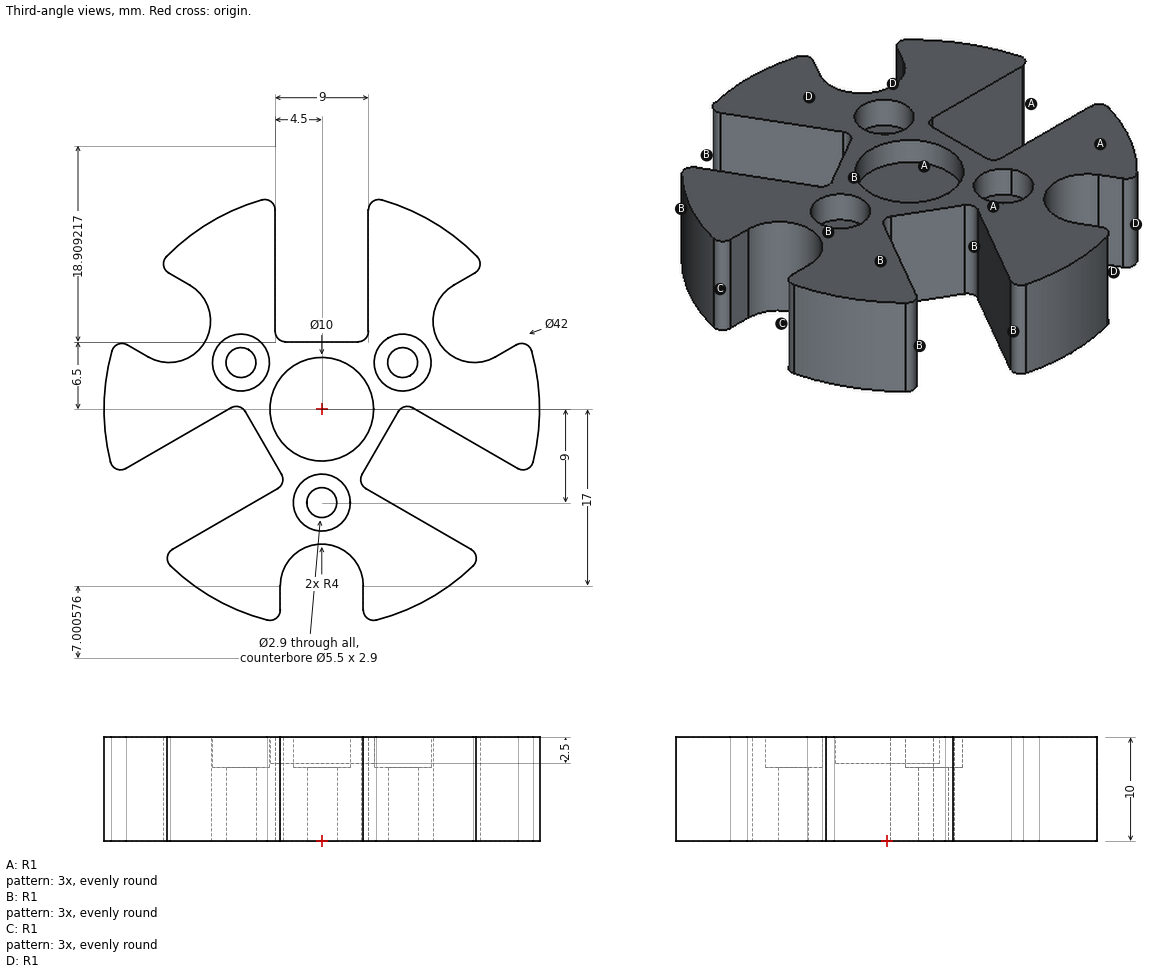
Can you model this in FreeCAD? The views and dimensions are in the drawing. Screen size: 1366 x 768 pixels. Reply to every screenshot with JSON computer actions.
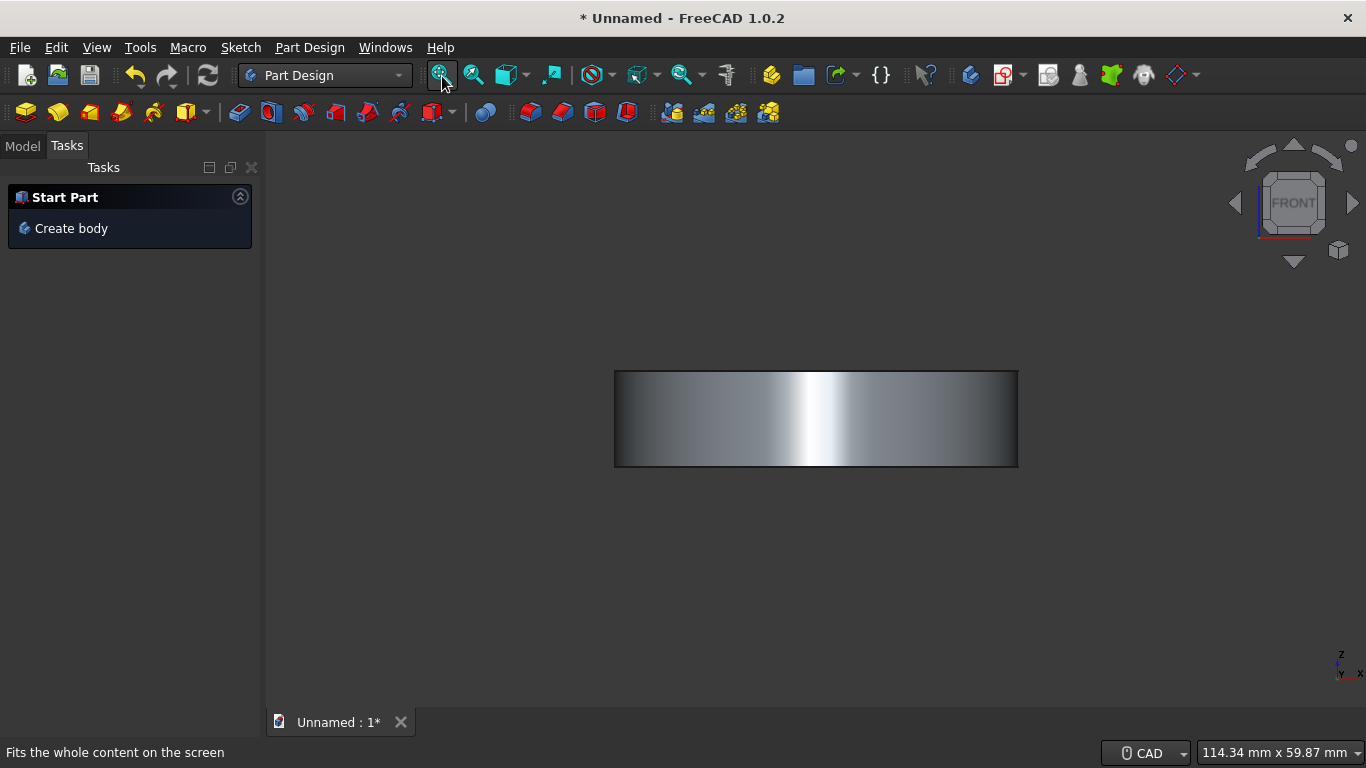
{"action": "key", "text": "3"}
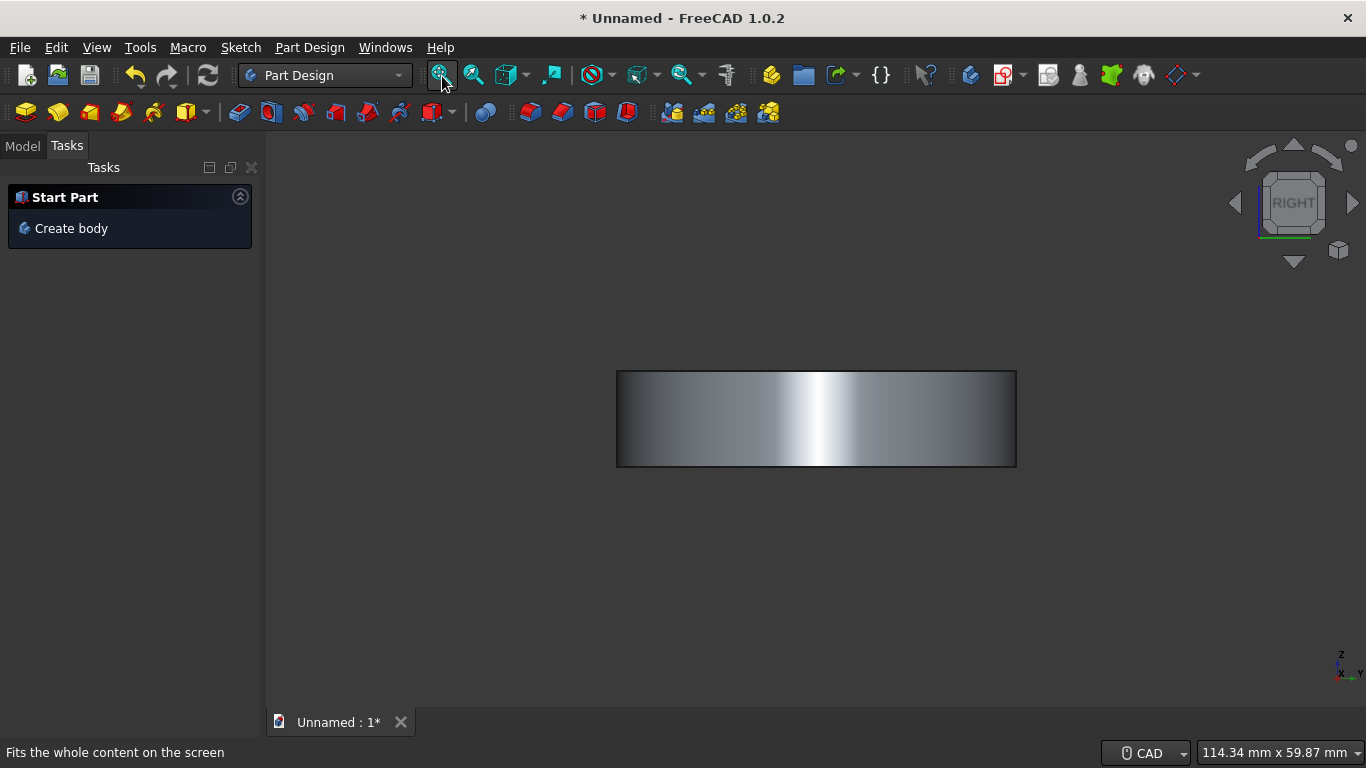
{"action": "left_click", "coordinate": [442, 76]}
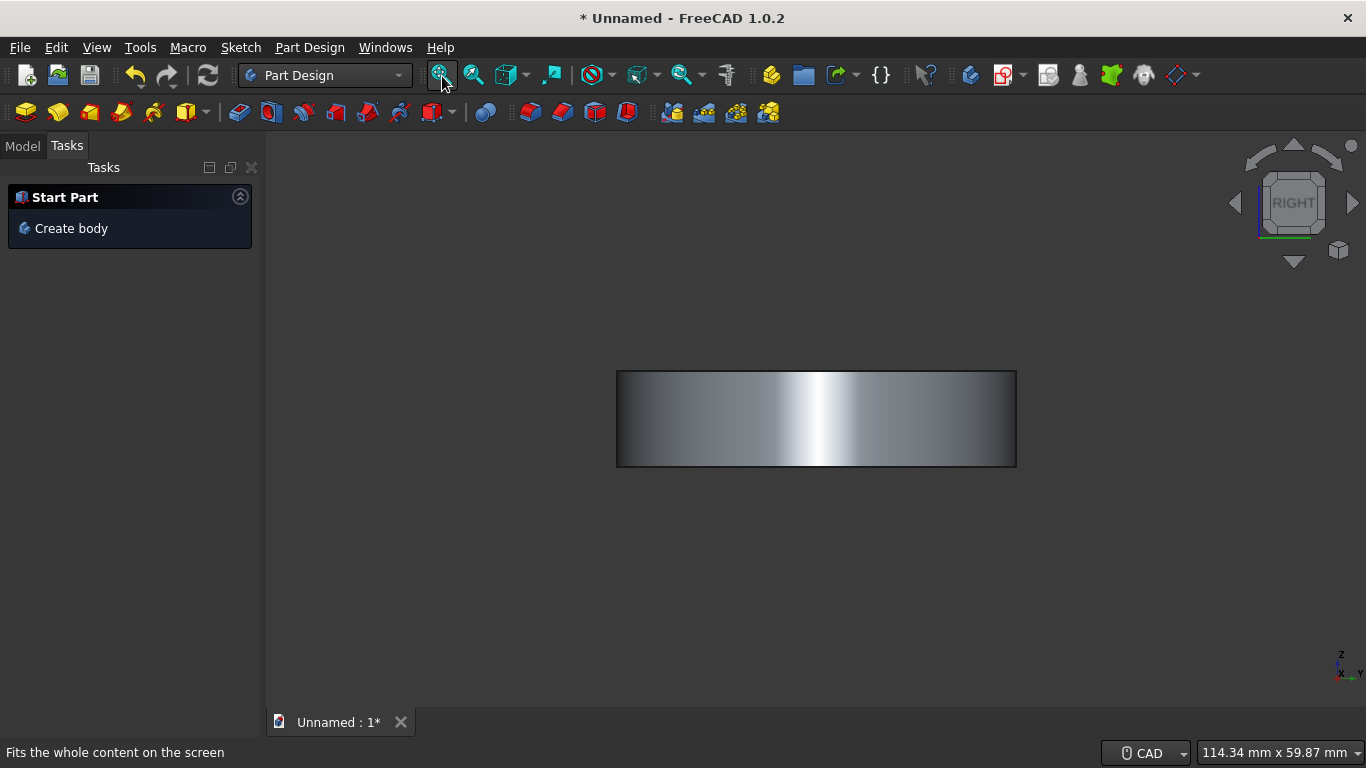
{"action": "key", "text": "5"}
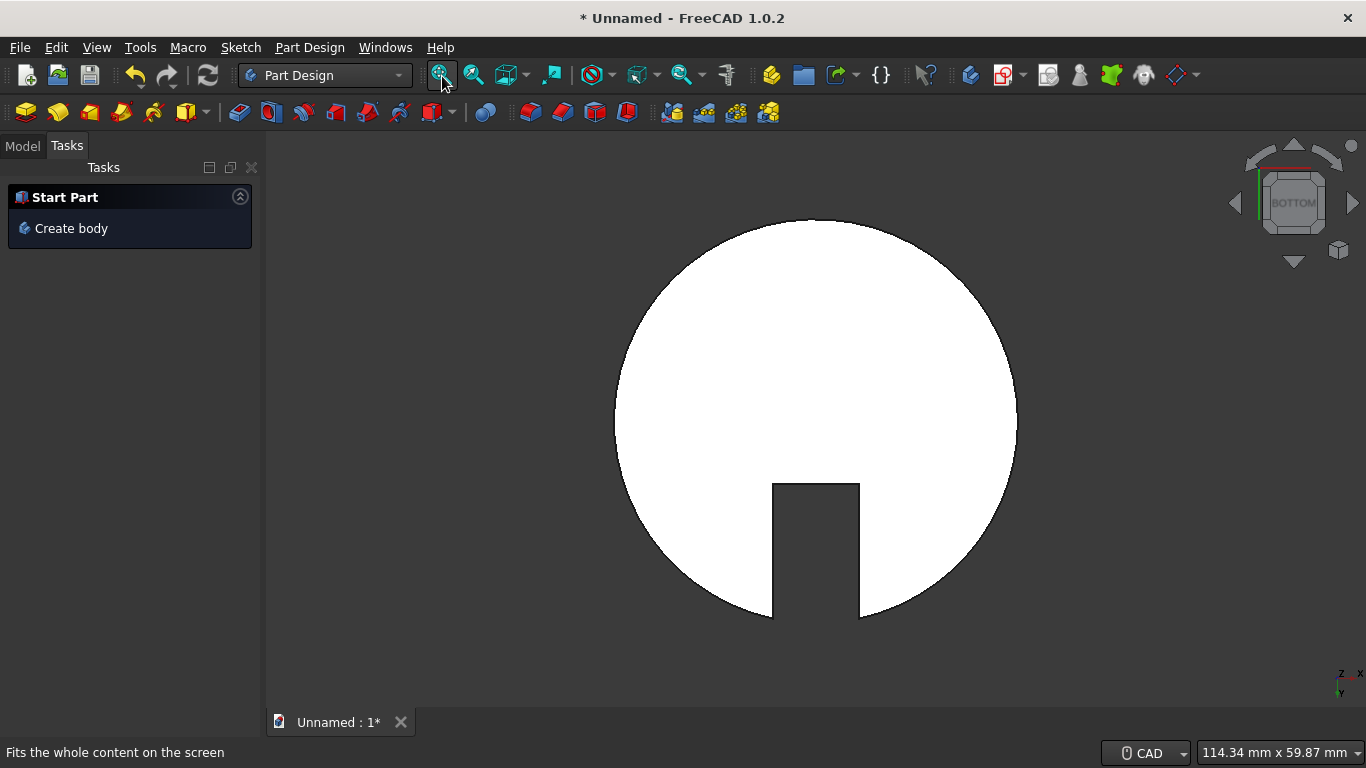
{"action": "key", "text": "4"}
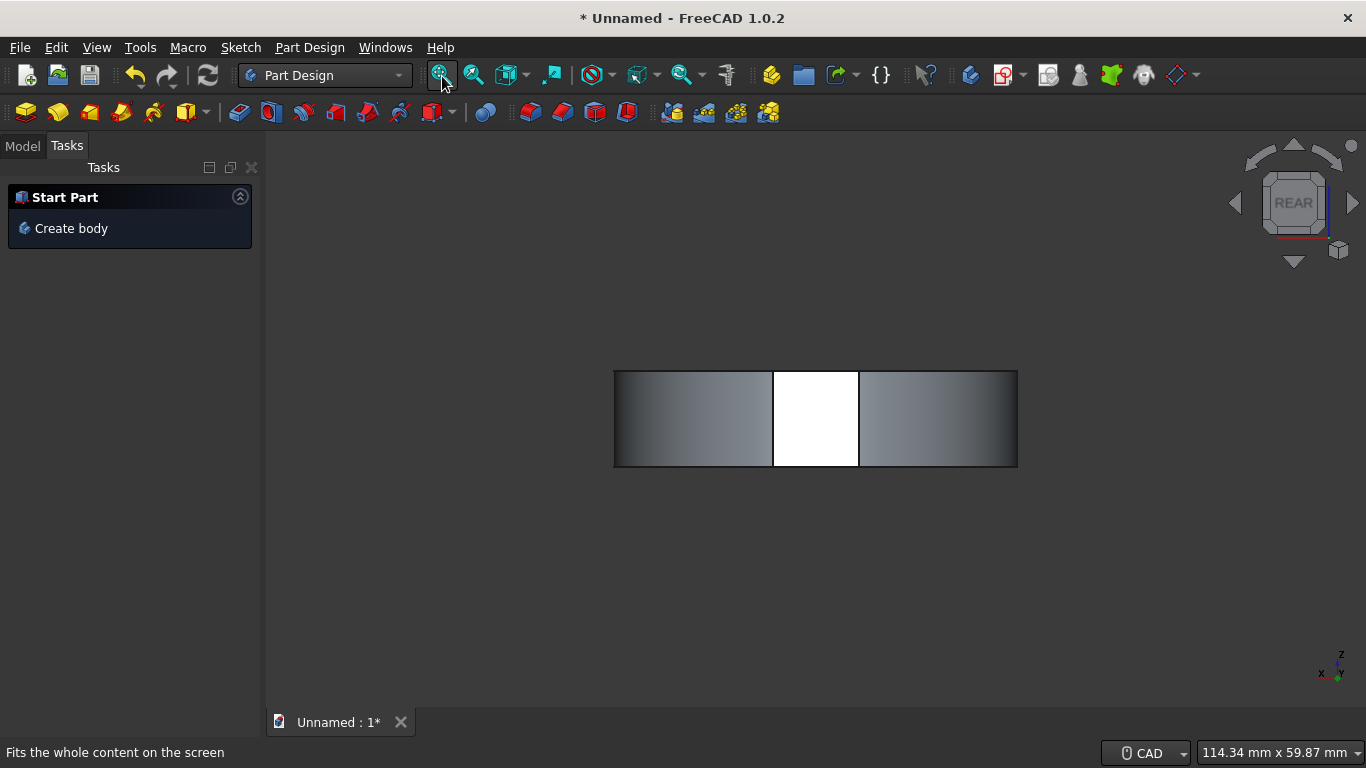
{"action": "left_click", "coordinate": [442, 76]}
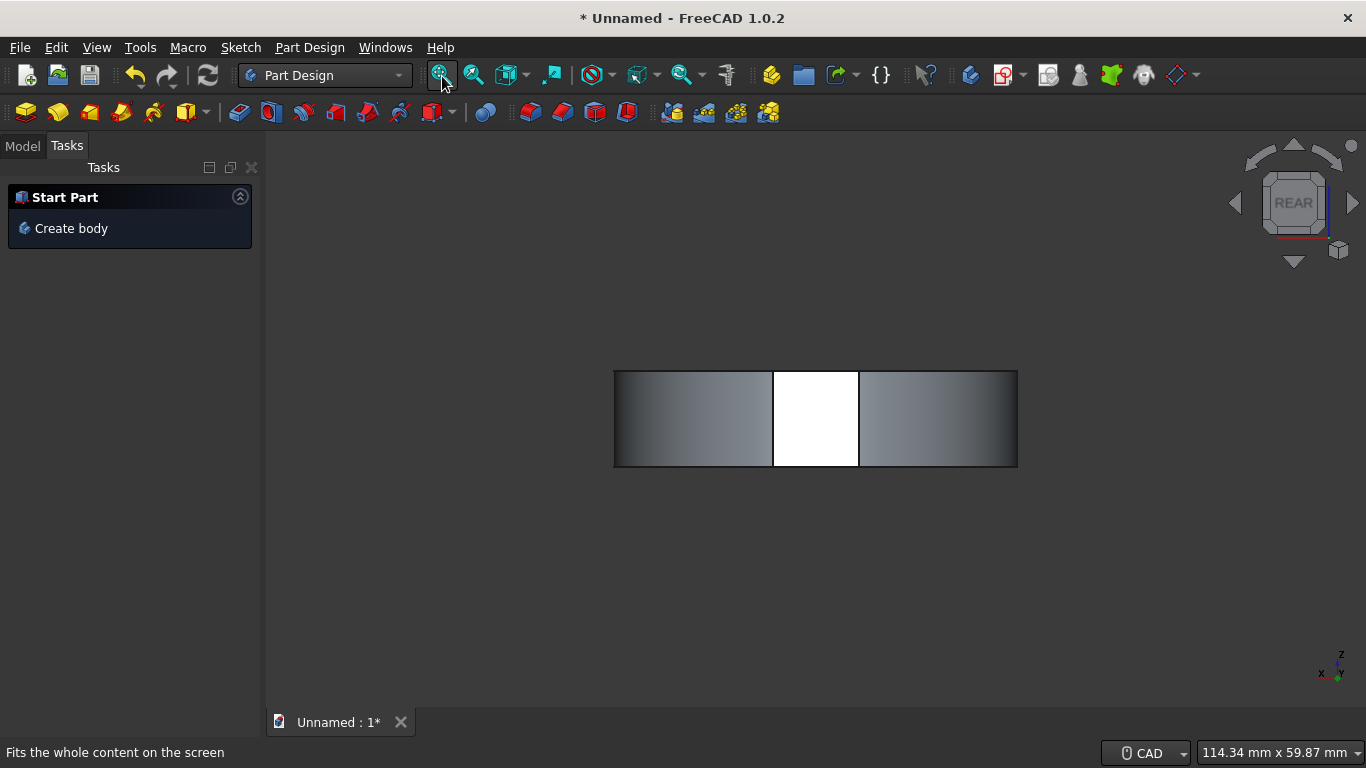
{"action": "left_click", "coordinate": [859, 418]}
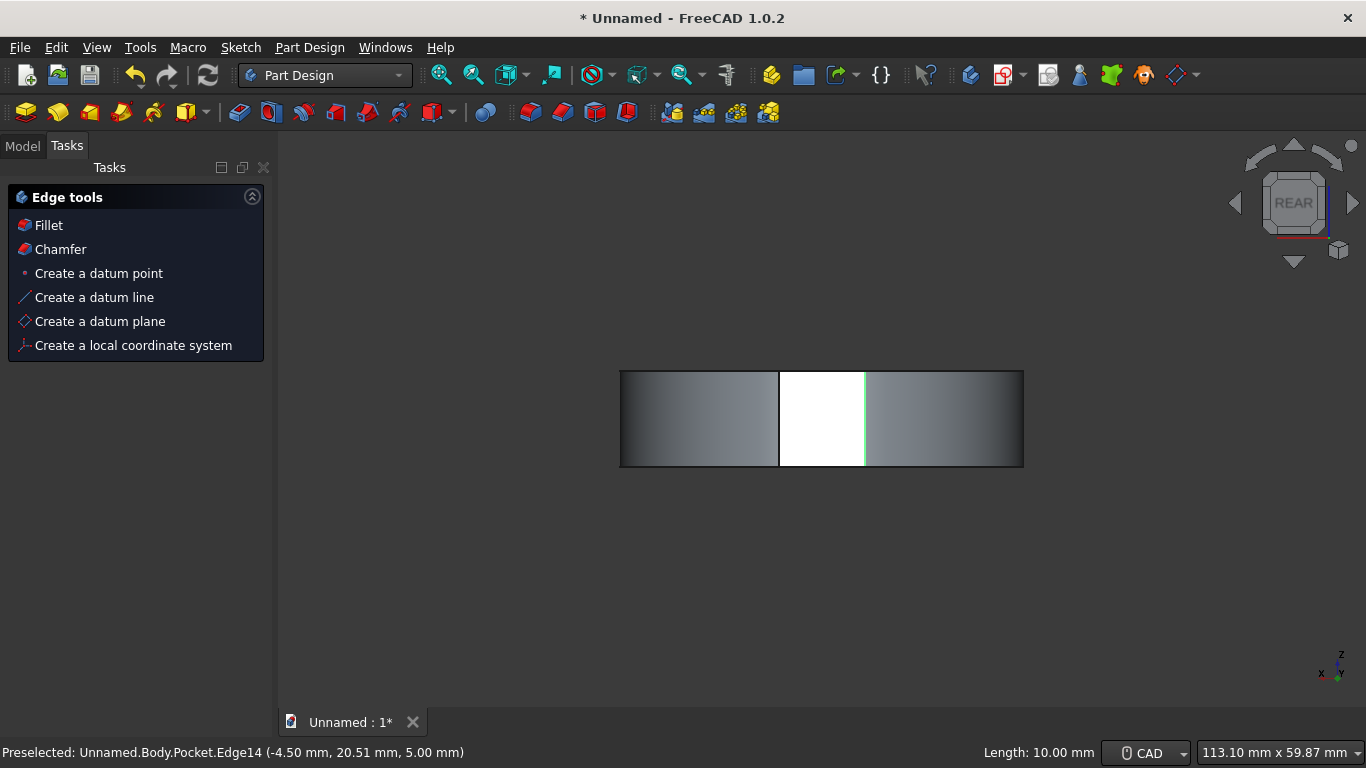
{"action": "left_click", "coordinate": [779, 418], "text": "ctrl"}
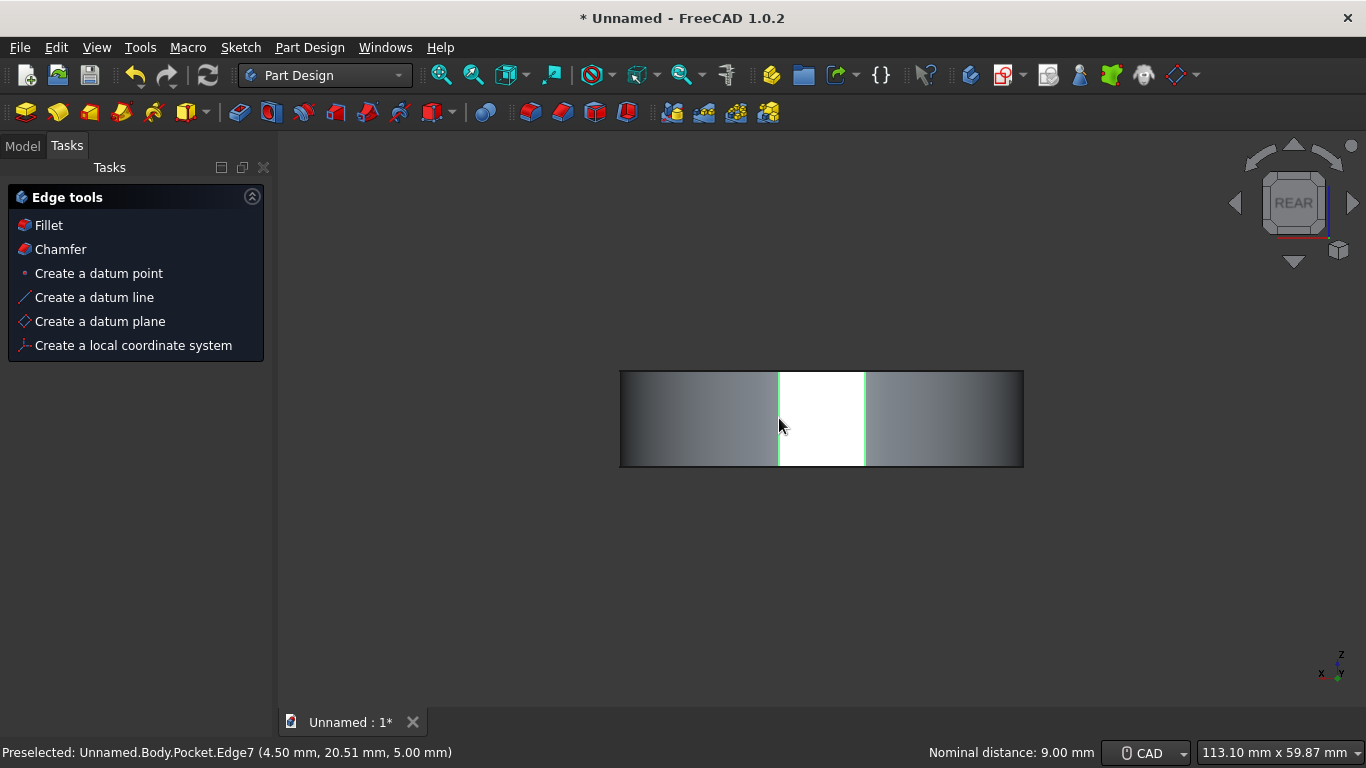
{"action": "key", "text": "6"}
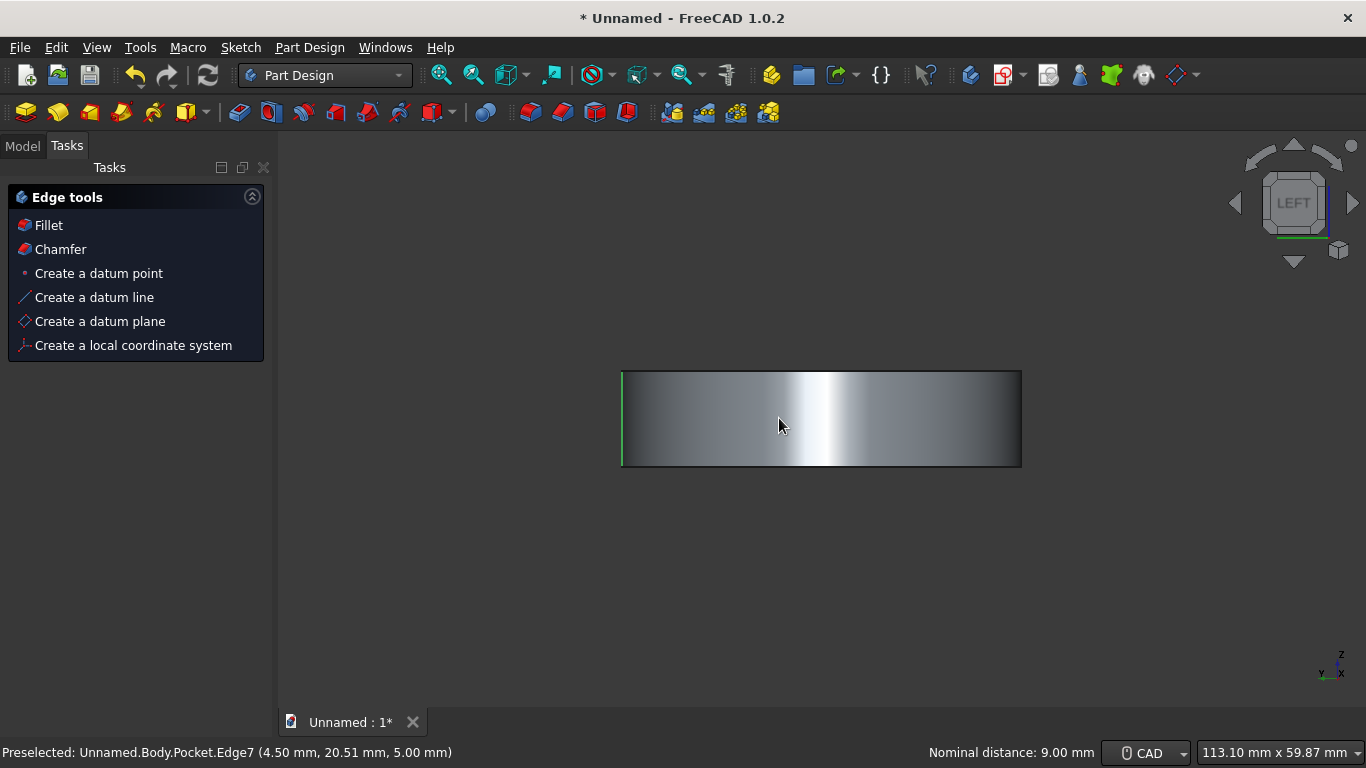
{"action": "left_click", "coordinate": [442, 76]}